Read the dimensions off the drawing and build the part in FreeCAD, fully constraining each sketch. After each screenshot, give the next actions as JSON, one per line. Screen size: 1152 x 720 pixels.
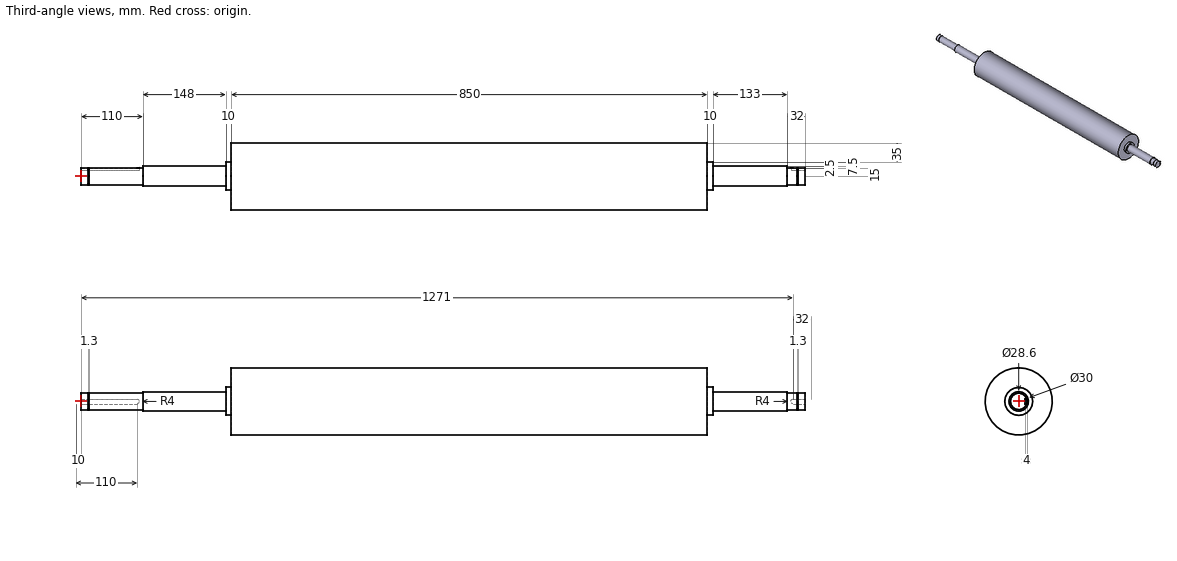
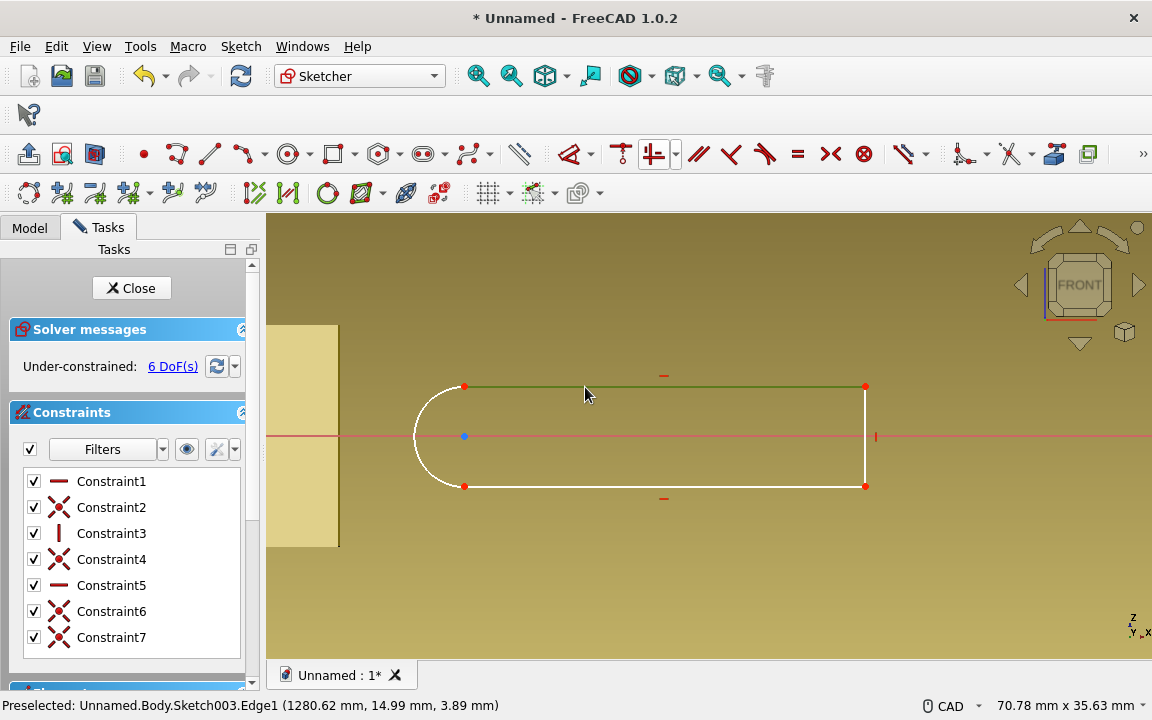
{"action": "left_click", "coordinate": [424, 407]}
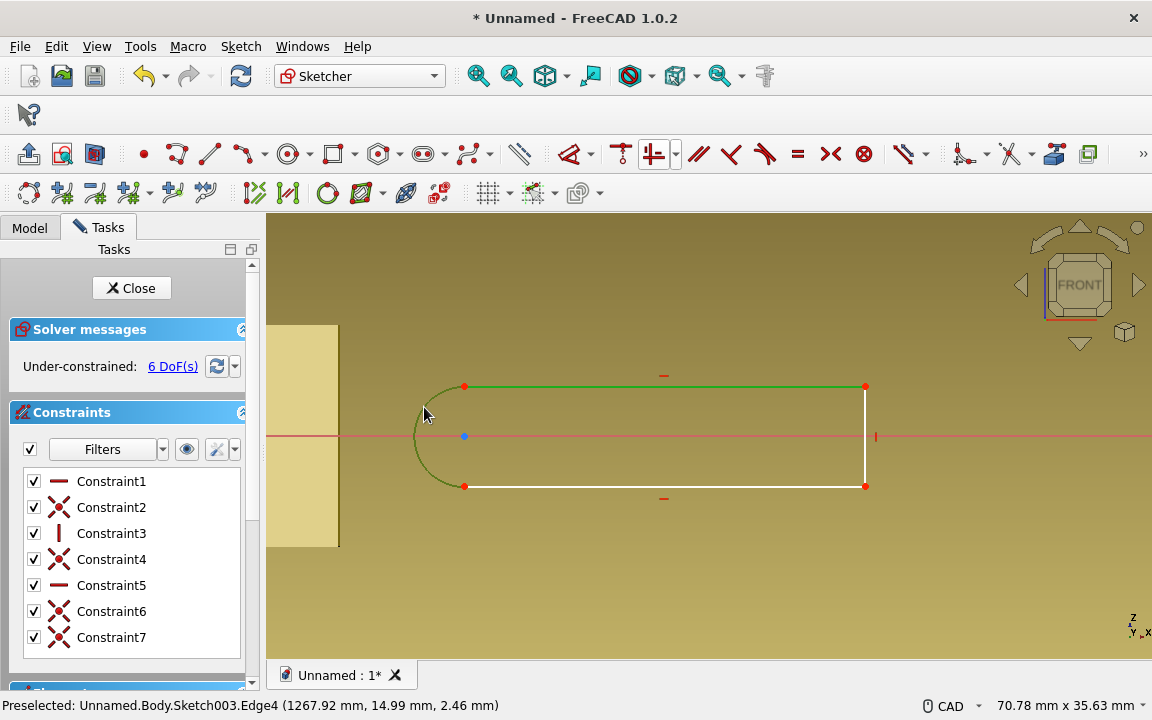
{"action": "left_click", "coordinate": [765, 154]}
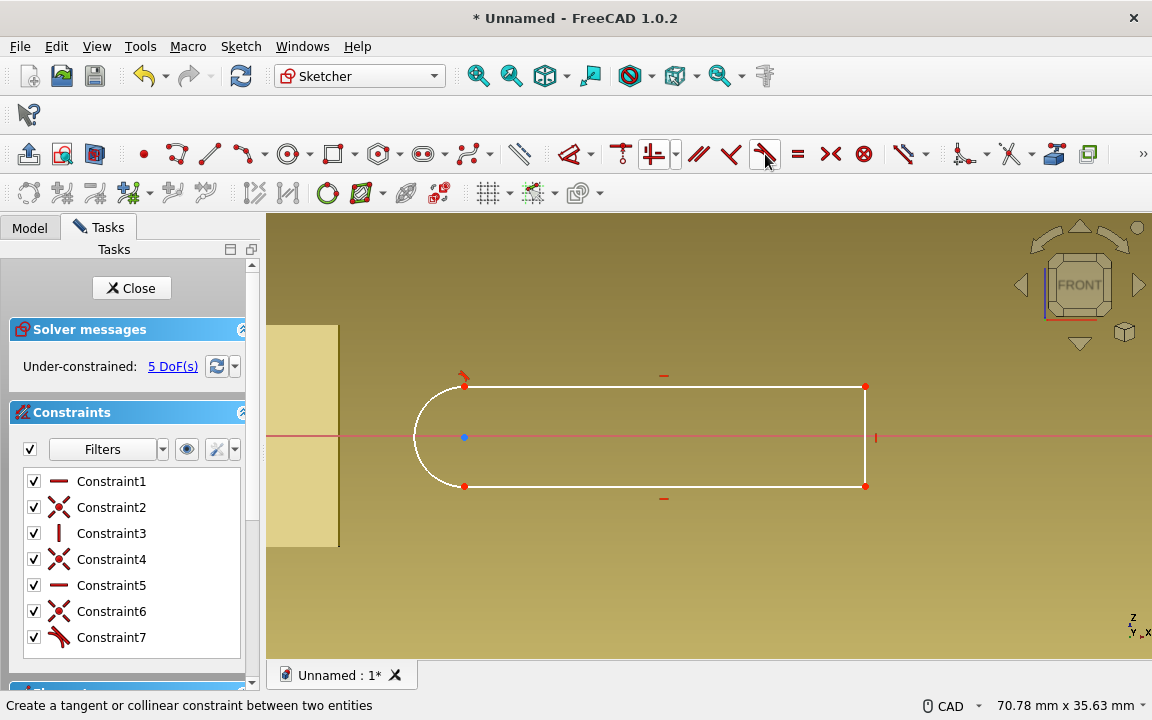
{"action": "left_click", "coordinate": [745, 487]}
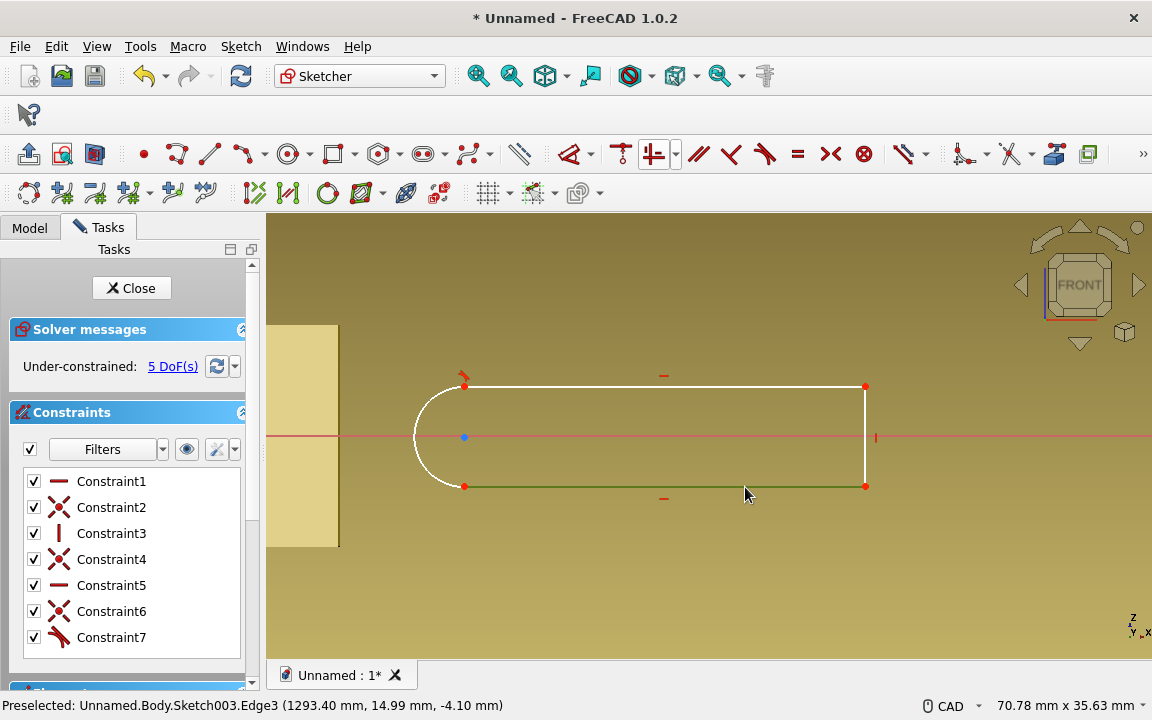
{"action": "left_click", "coordinate": [424, 408]}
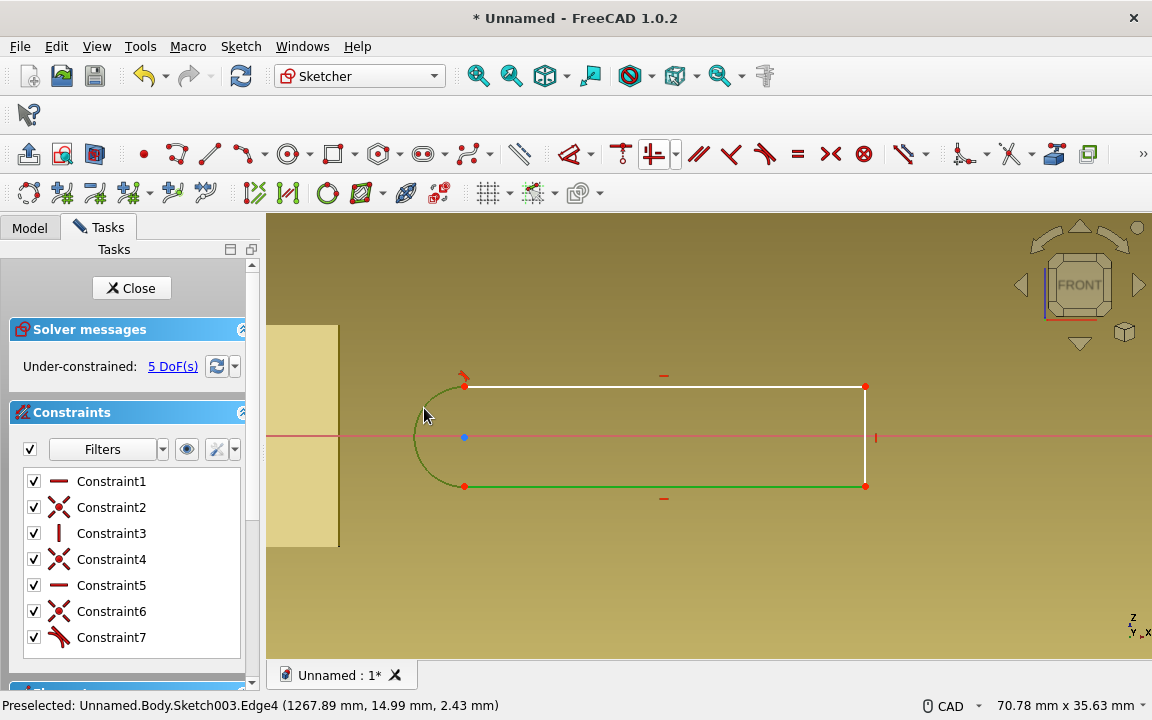
{"action": "key", "text": "t"}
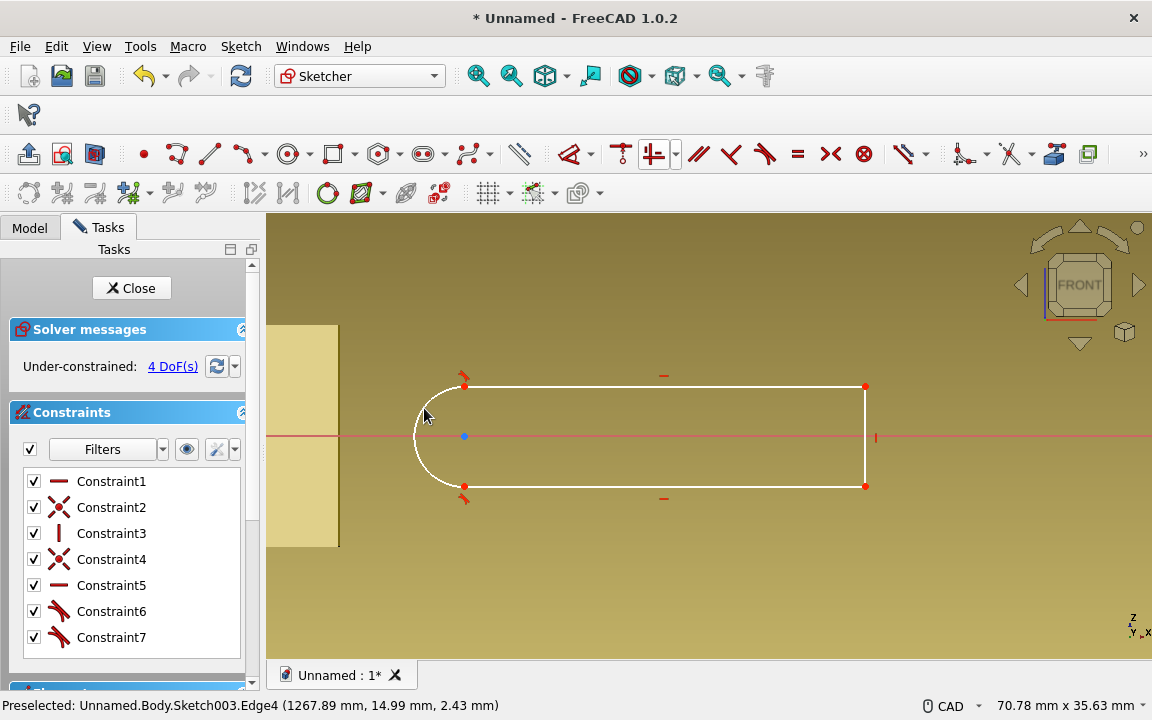
{"action": "left_click", "coordinate": [464, 437]}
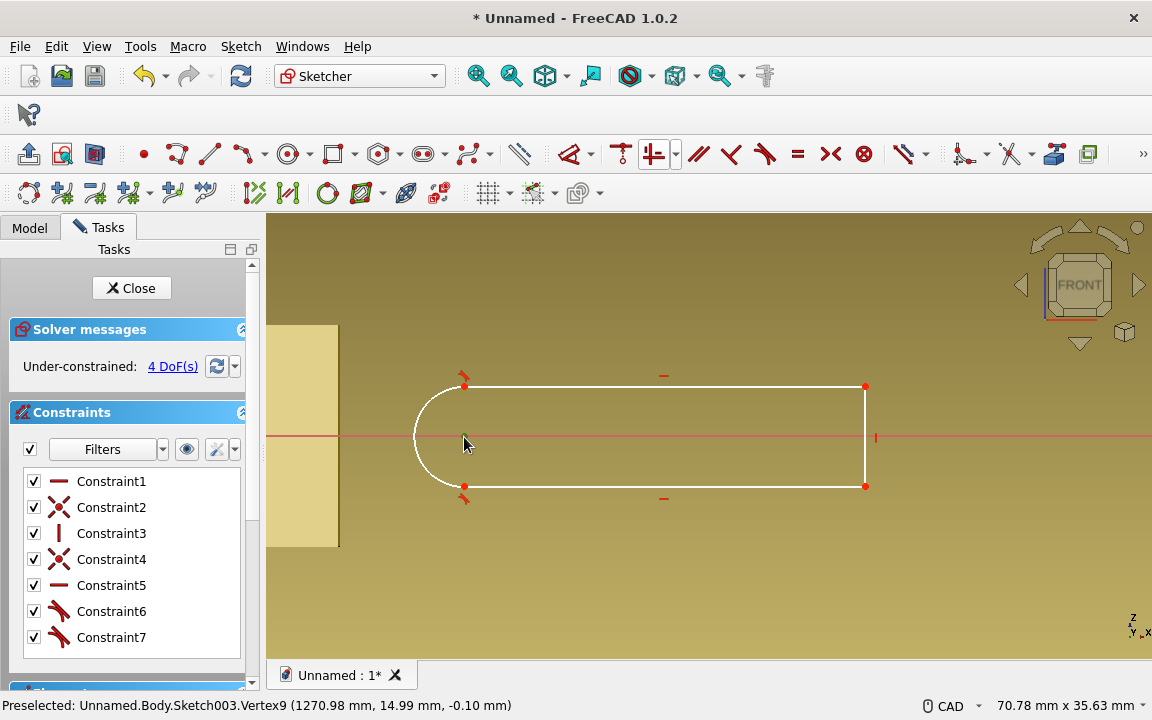
{"action": "left_click", "coordinate": [343, 436]}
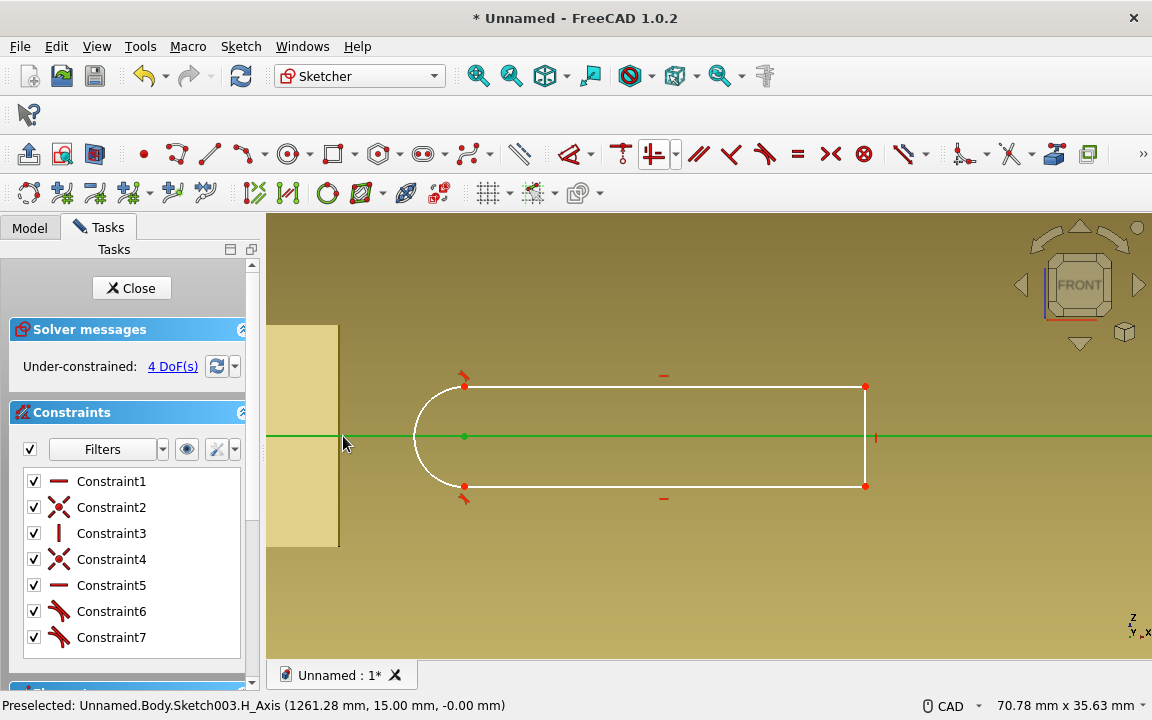
{"action": "key", "text": "c"}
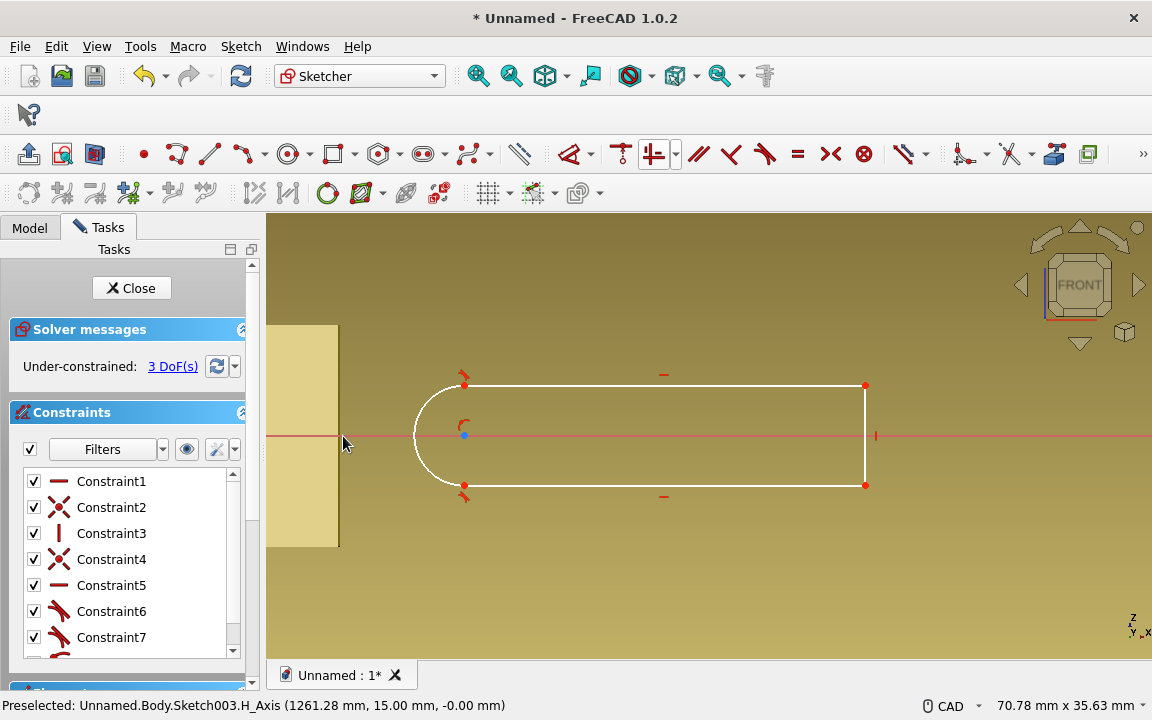
{"action": "key", "text": "d"}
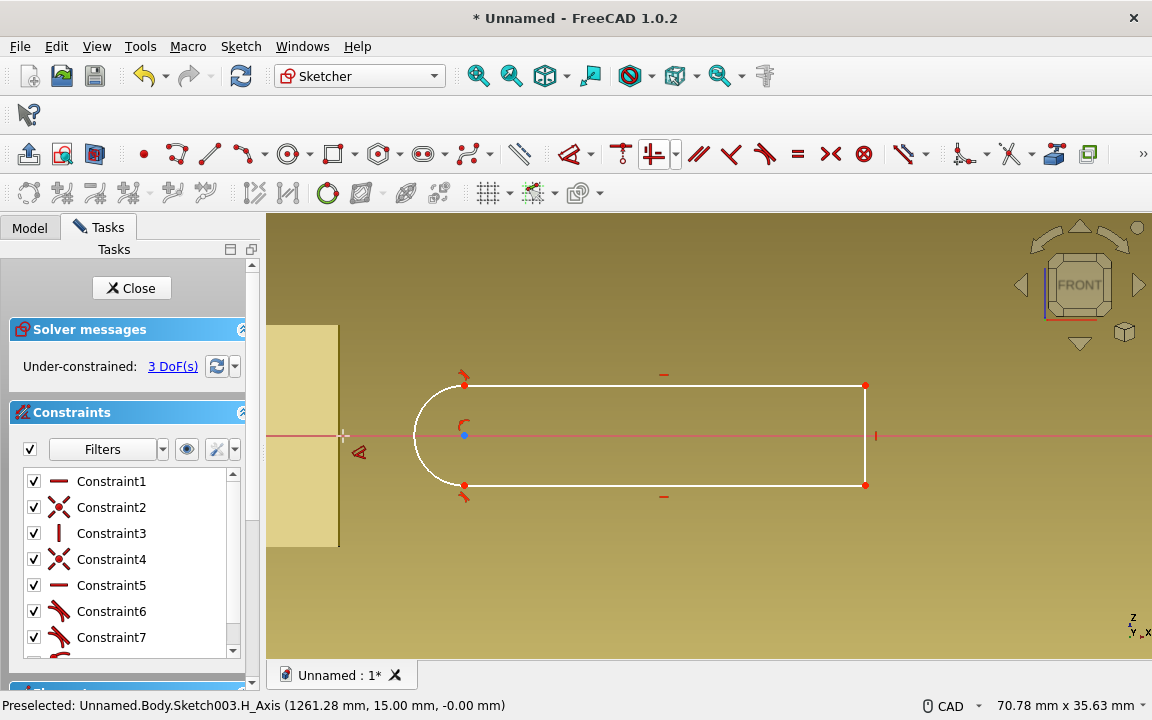
{"action": "left_click", "coordinate": [424, 406]}
{"action": "left_click", "coordinate": [398, 387]}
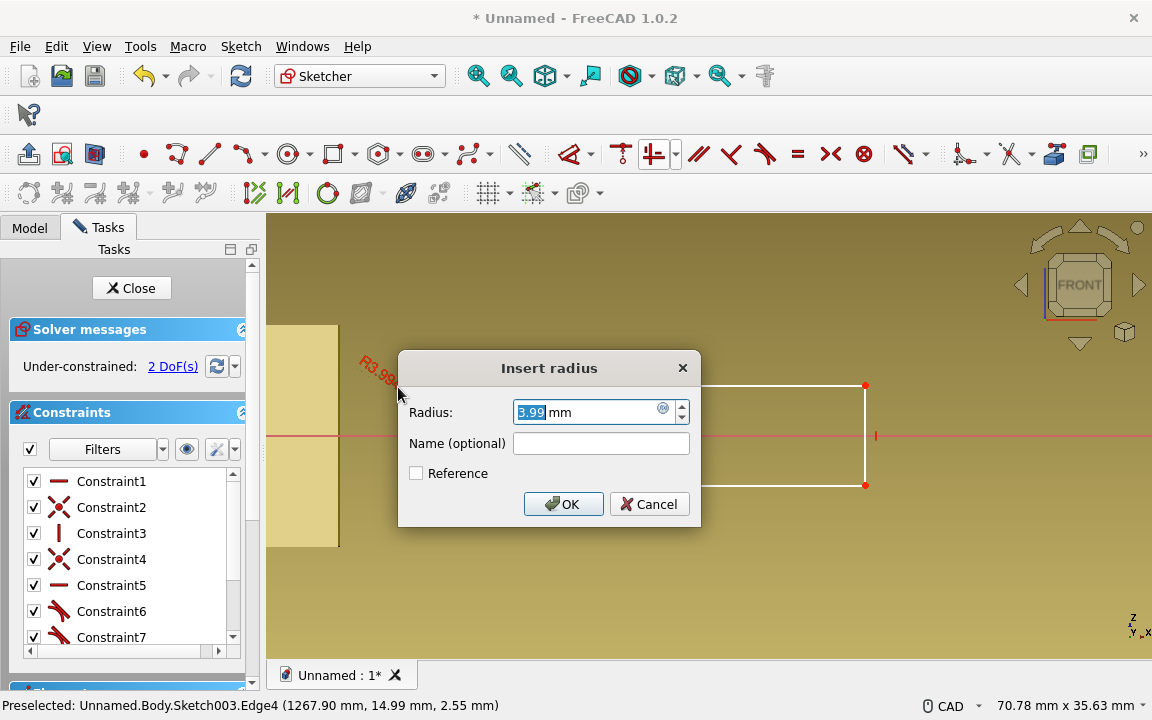
{"action": "type", "text": "4"}
{"action": "key", "text": "Return"}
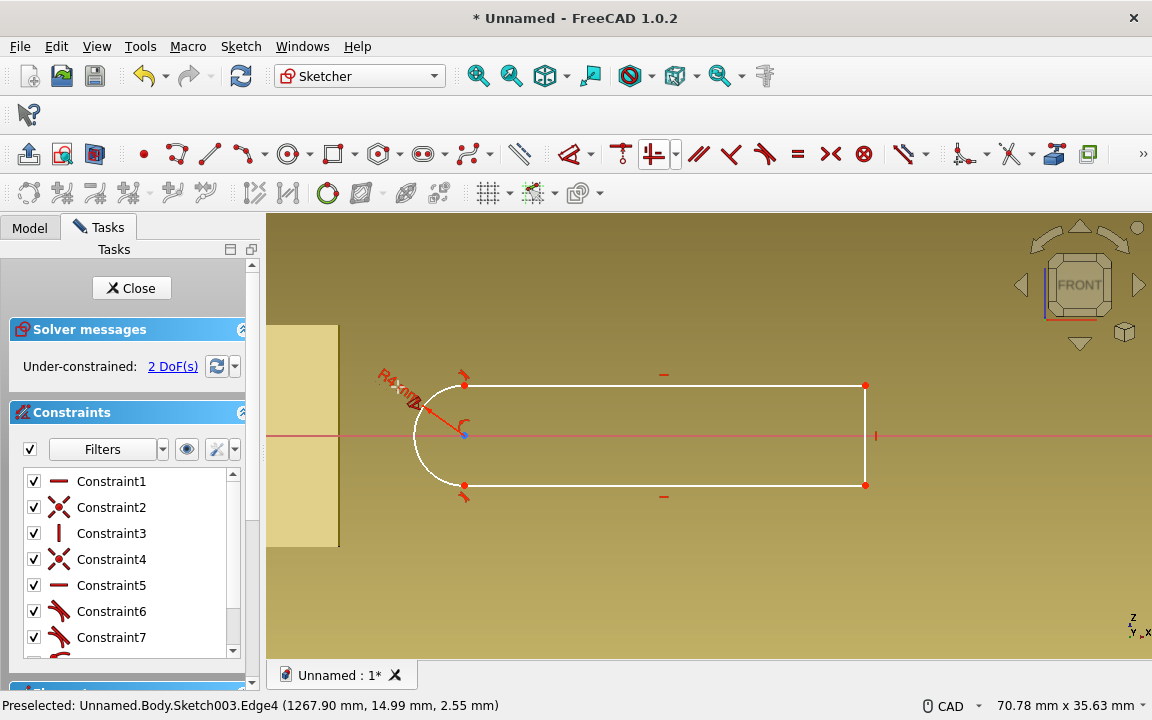
{"action": "left_click", "coordinate": [585, 386]}
{"action": "left_click", "coordinate": [665, 352]}